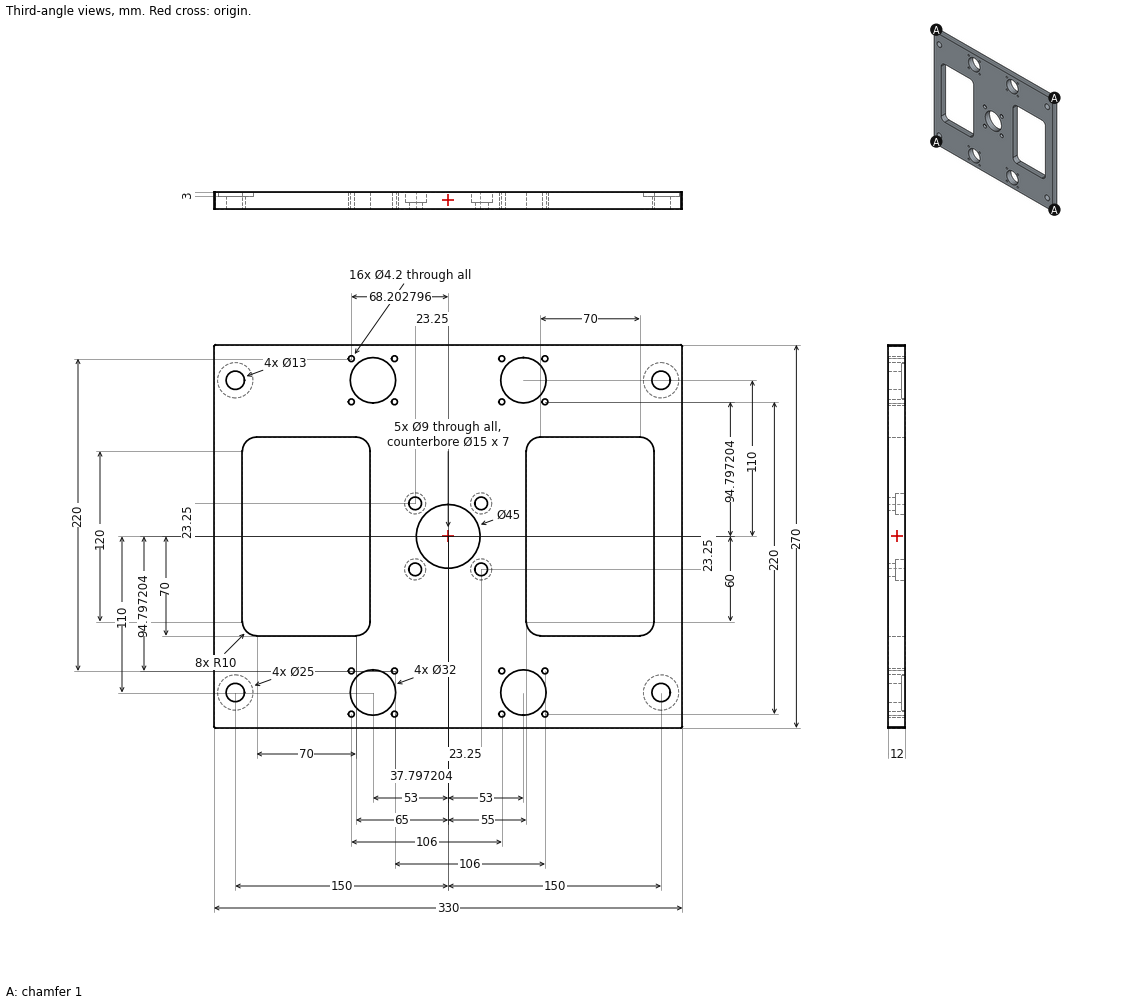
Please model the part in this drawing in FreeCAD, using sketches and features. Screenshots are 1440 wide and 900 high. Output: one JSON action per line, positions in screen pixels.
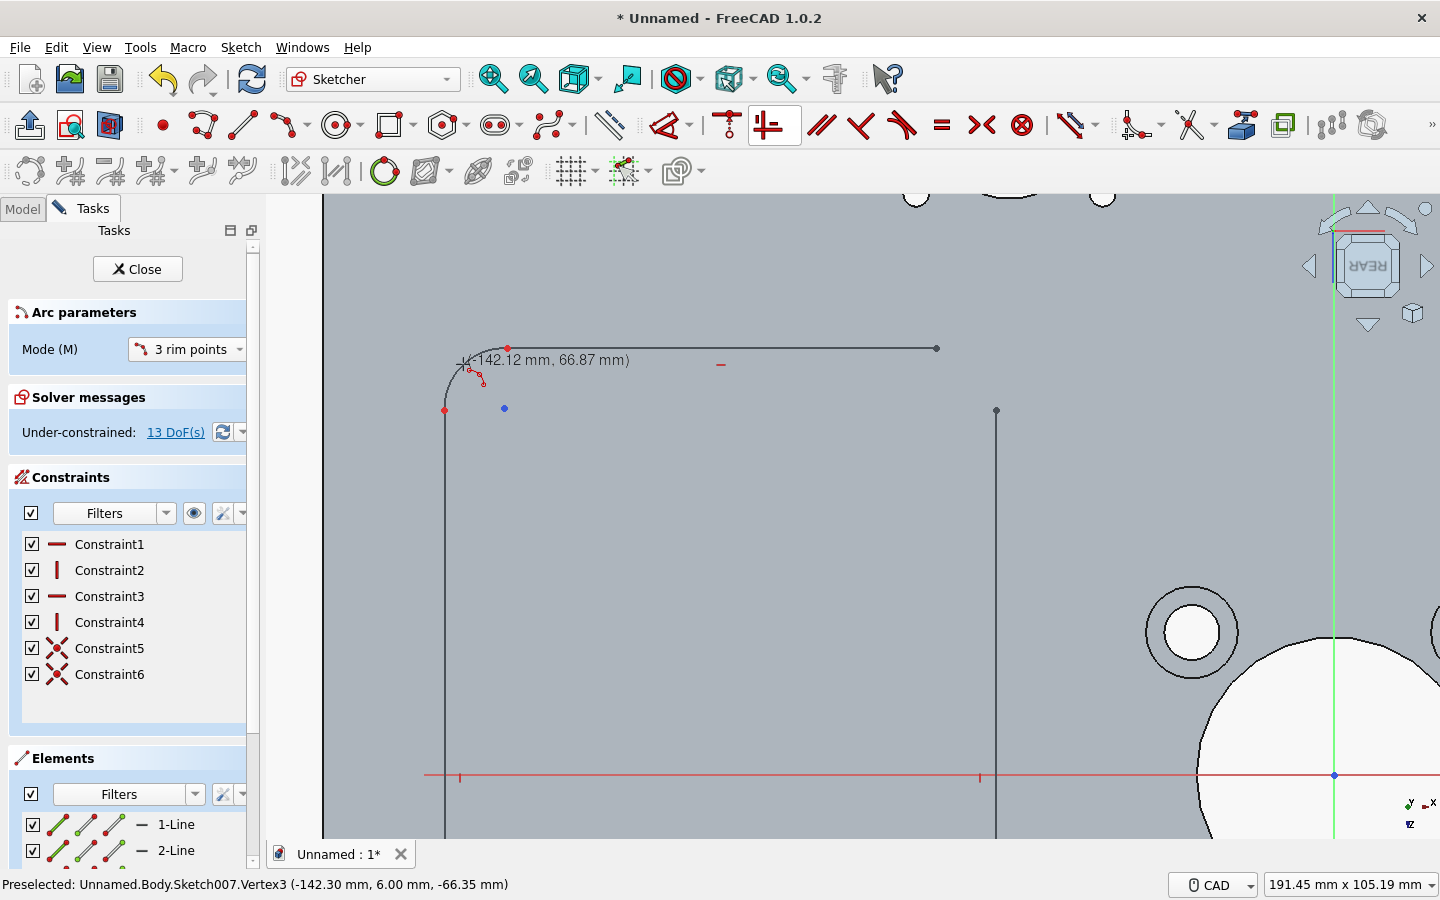
{"action": "scroll", "coordinate": [464, 366], "scroll_direction": "down", "scroll_amount": 5}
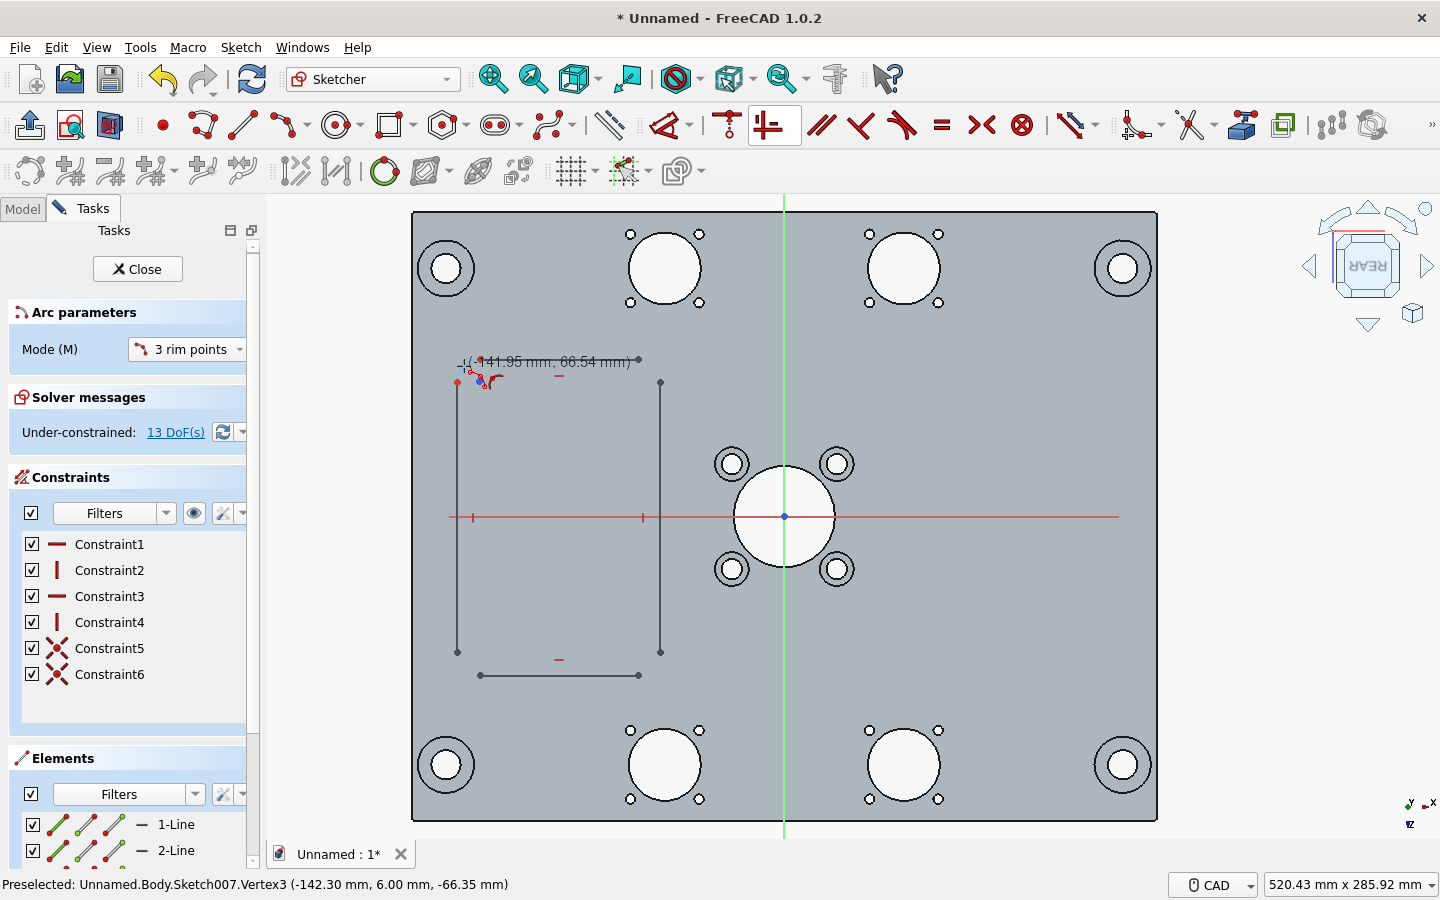
{"action": "left_click", "coordinate": [457, 653]}
{"action": "left_click", "coordinate": [480, 676]}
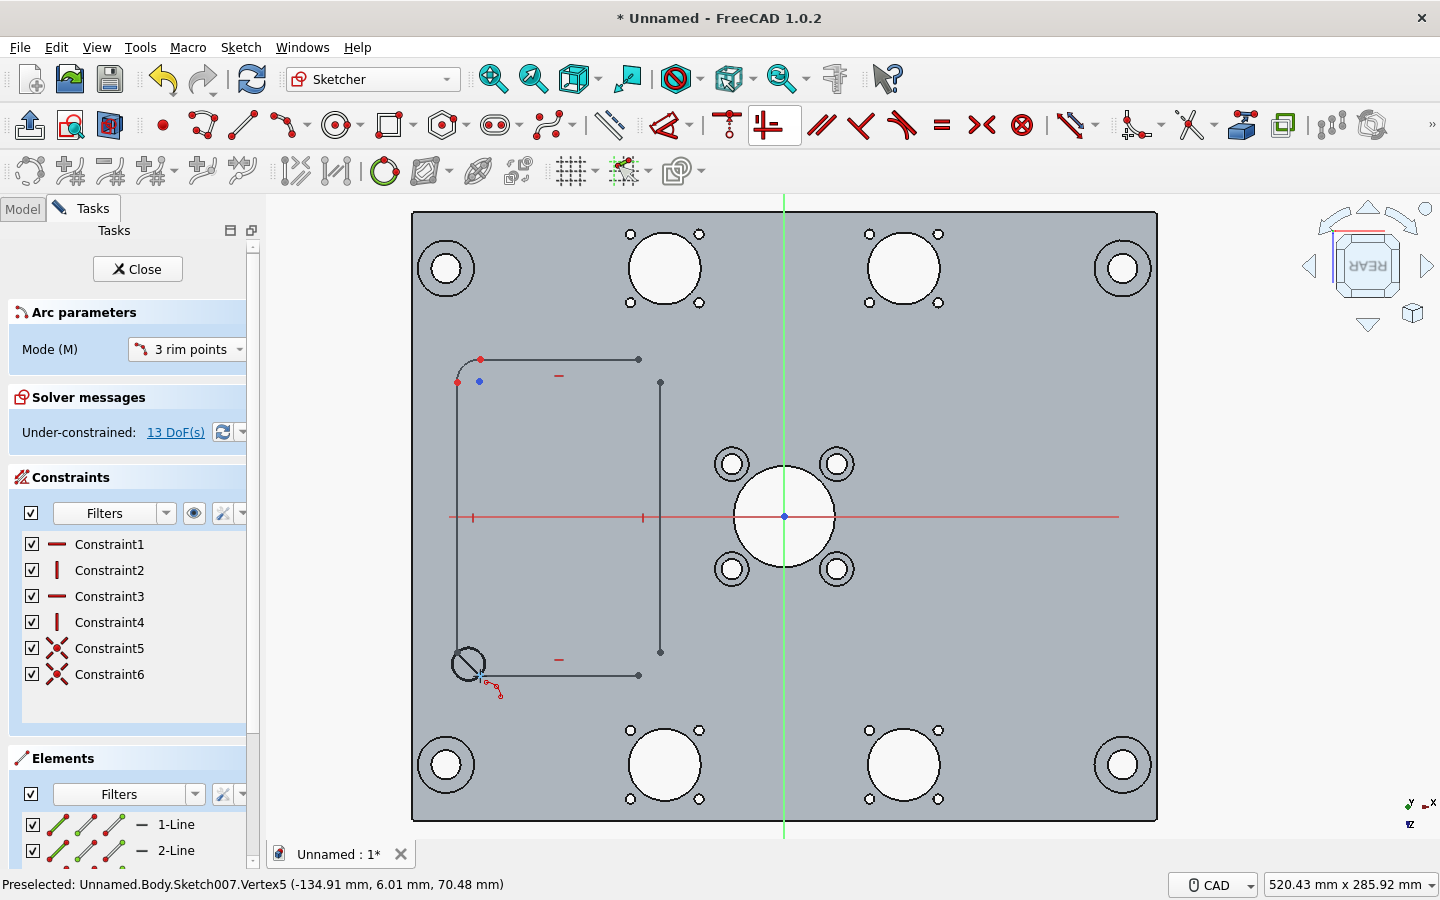
{"action": "scroll", "coordinate": [464, 668], "scroll_direction": "up", "scroll_amount": 5}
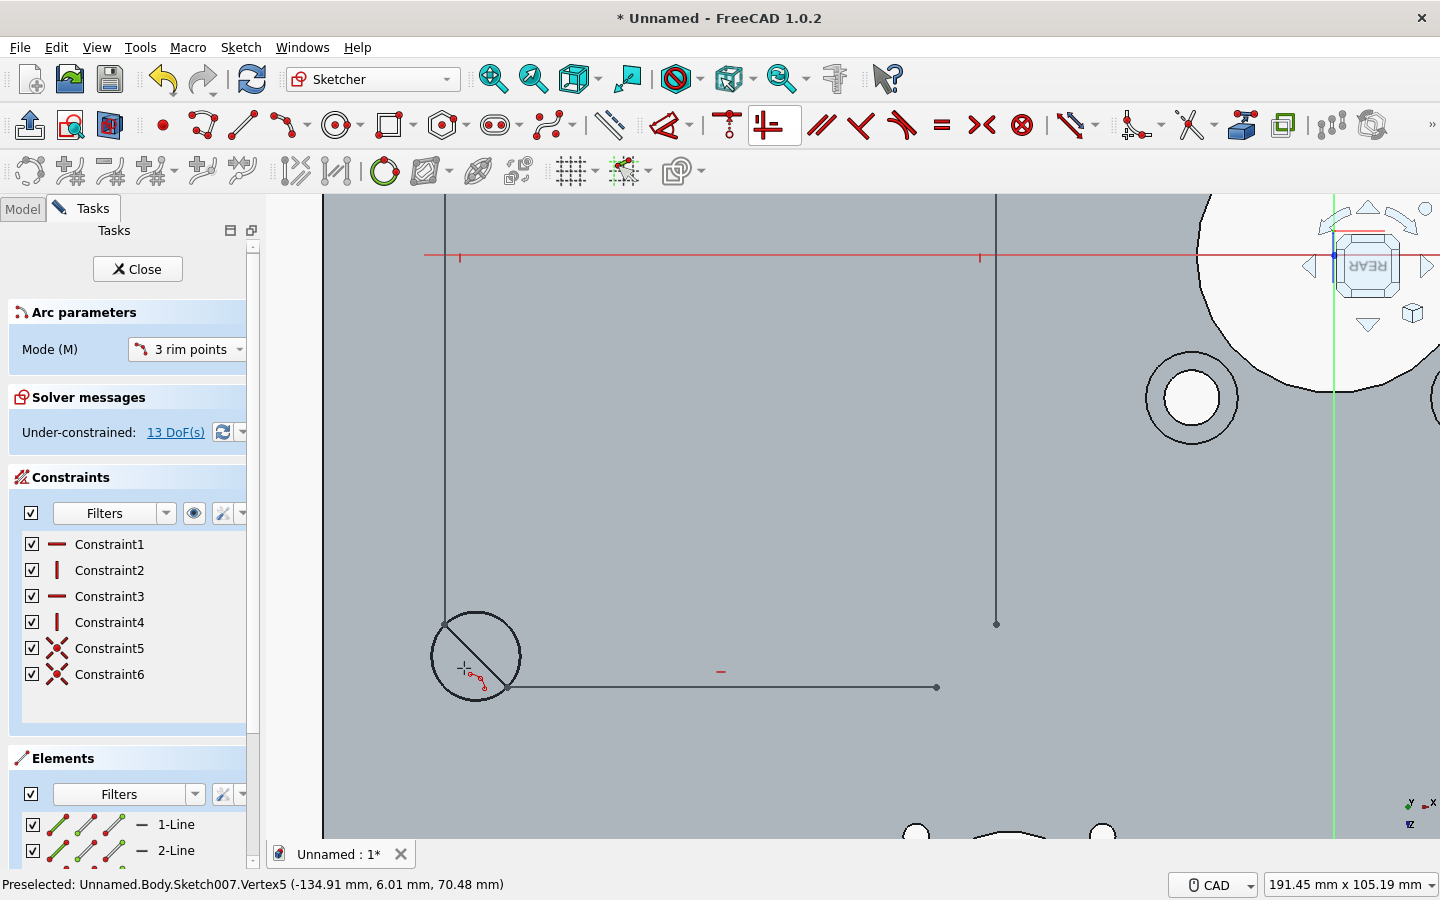
{"action": "left_click", "coordinate": [463, 667]}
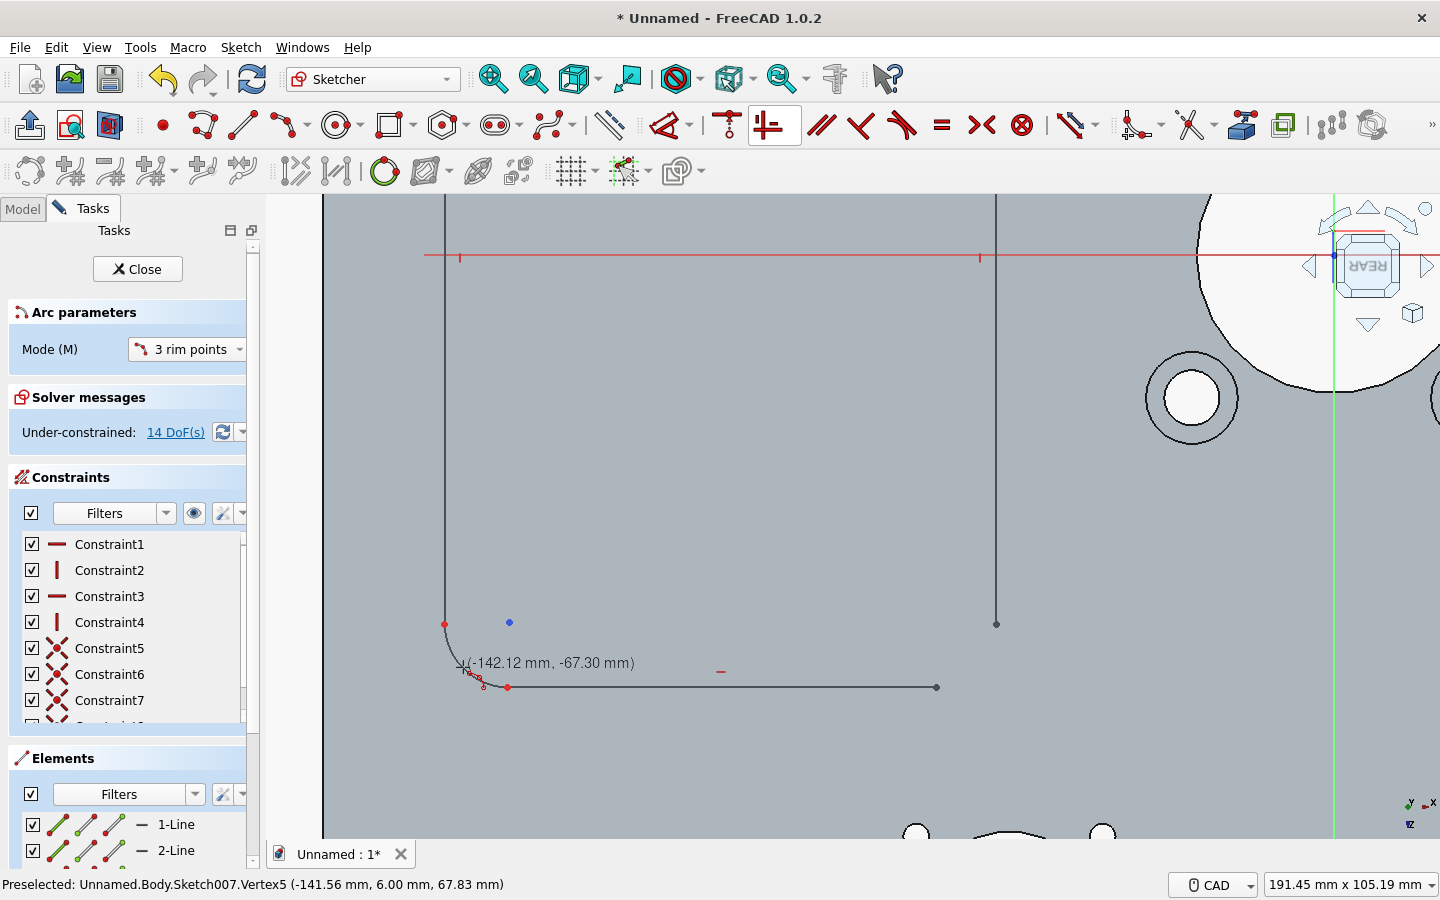
{"action": "left_click", "coordinate": [937, 687]}
{"action": "left_click", "coordinate": [996, 625]}
{"action": "left_click", "coordinate": [979, 667]}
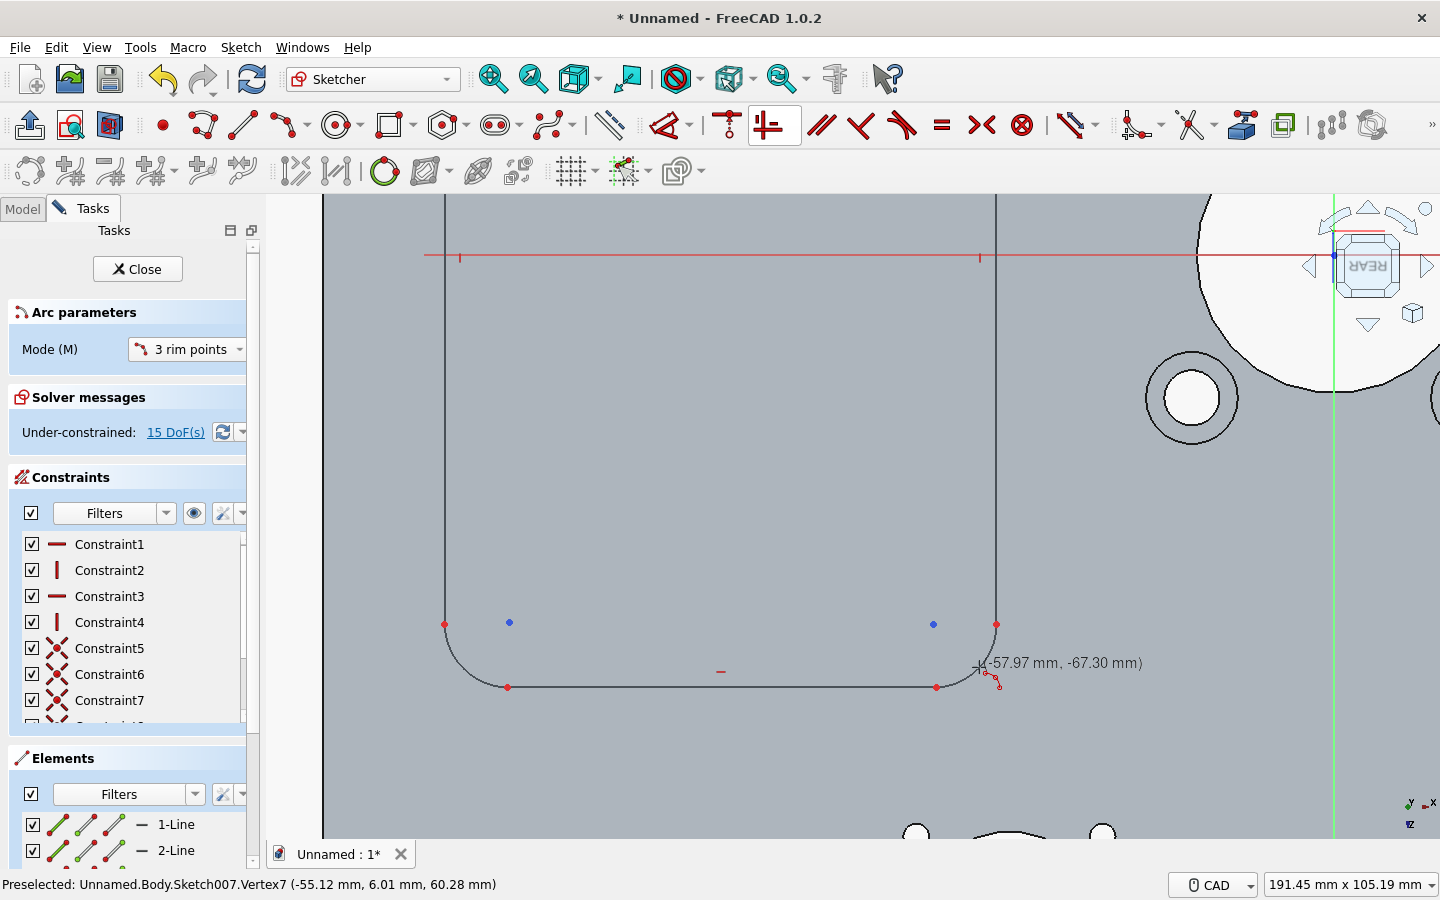
{"action": "scroll", "coordinate": [464, 669], "scroll_direction": "down", "scroll_amount": 5}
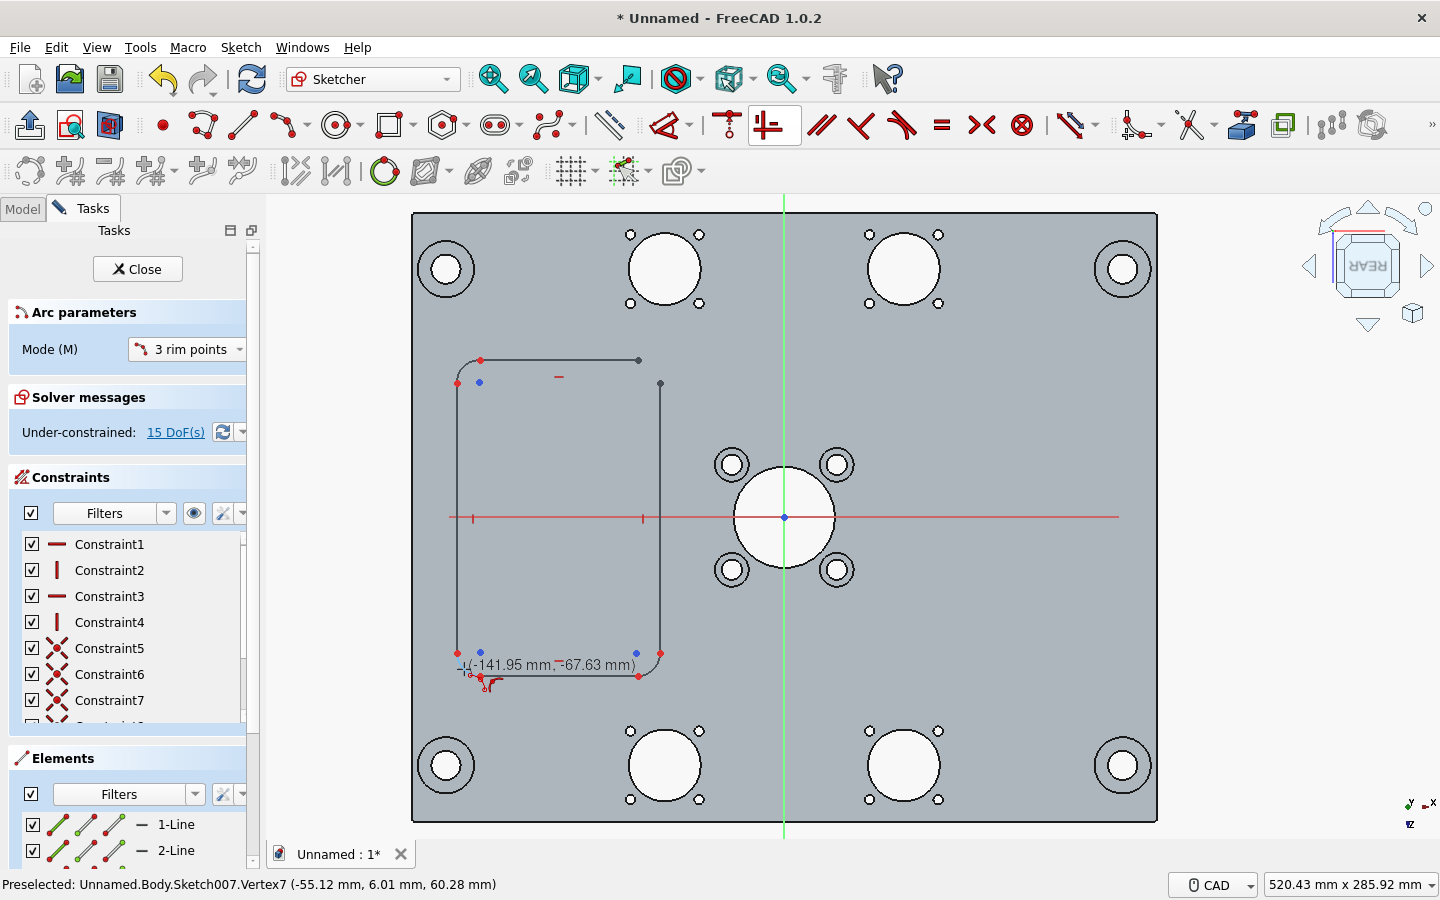
{"action": "left_click", "coordinate": [660, 383]}
{"action": "left_click", "coordinate": [638, 360]}